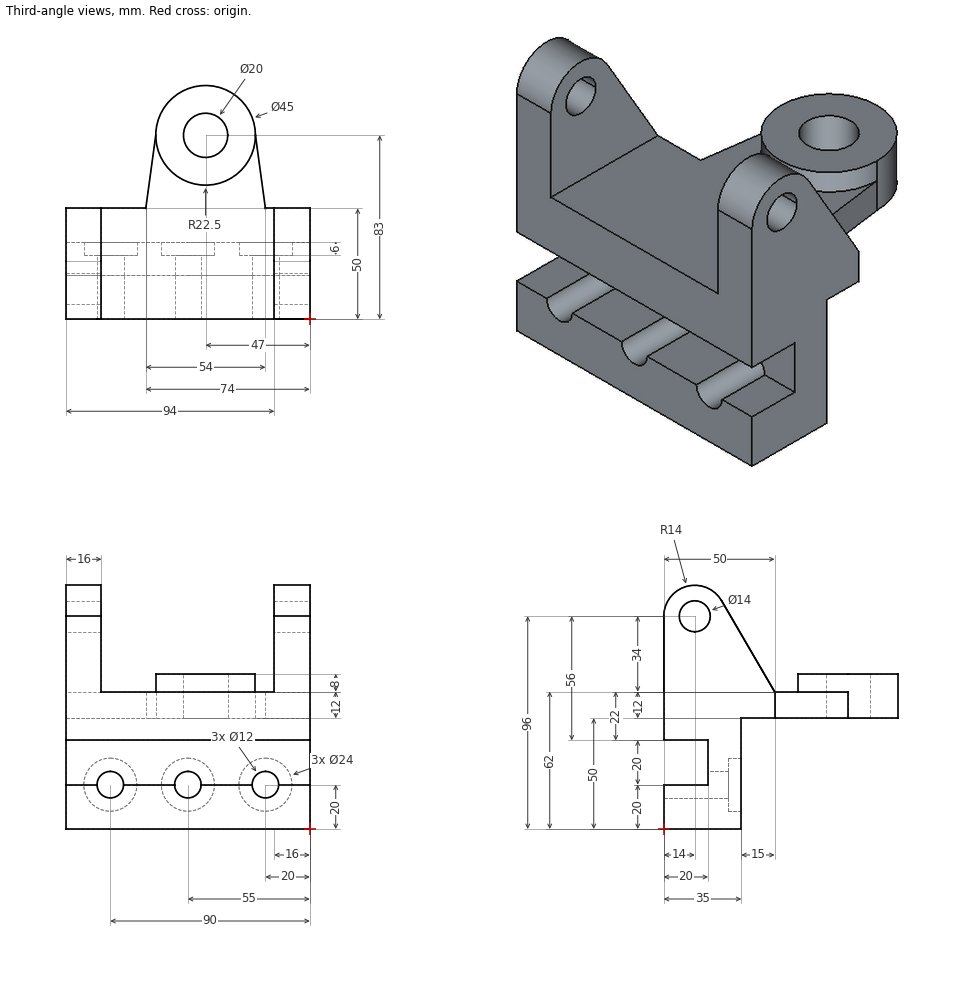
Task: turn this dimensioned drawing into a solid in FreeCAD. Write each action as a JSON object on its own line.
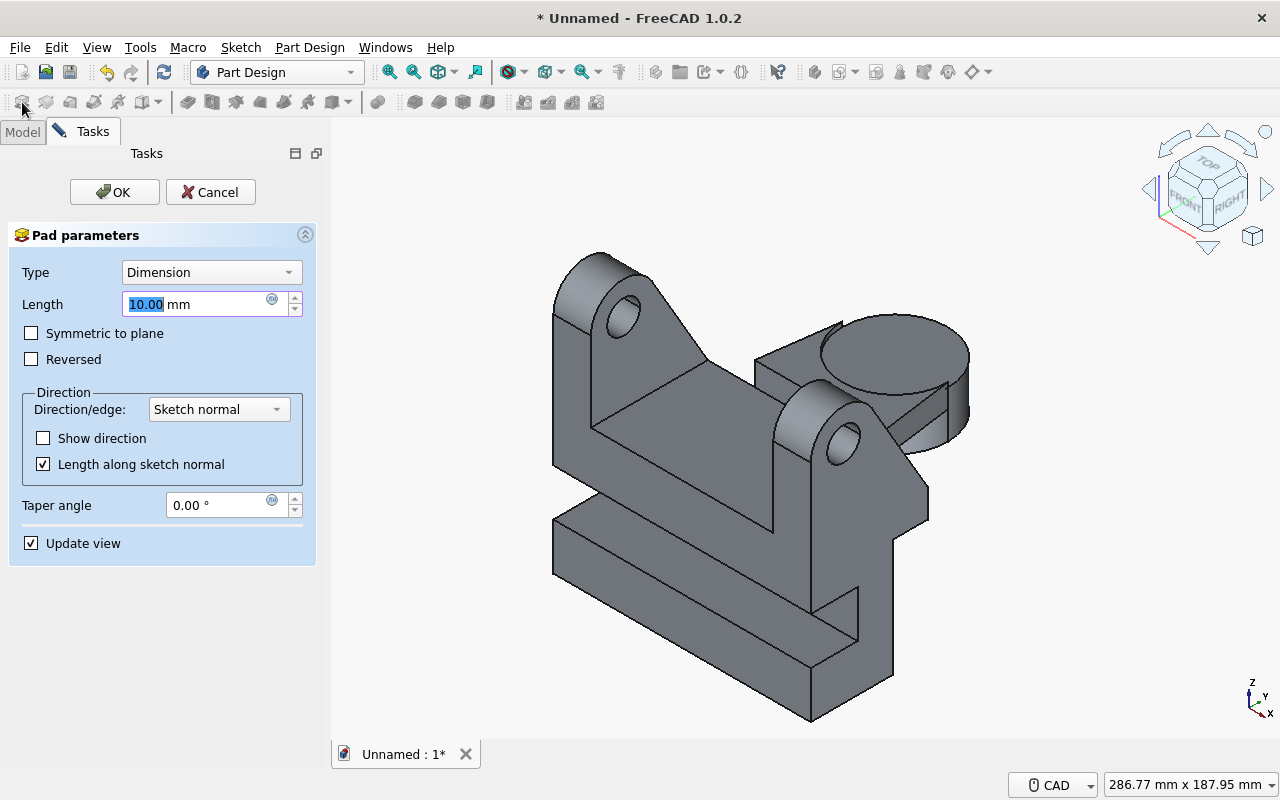
{"action": "type", "text": "12"}
{"action": "key", "text": "Tab"}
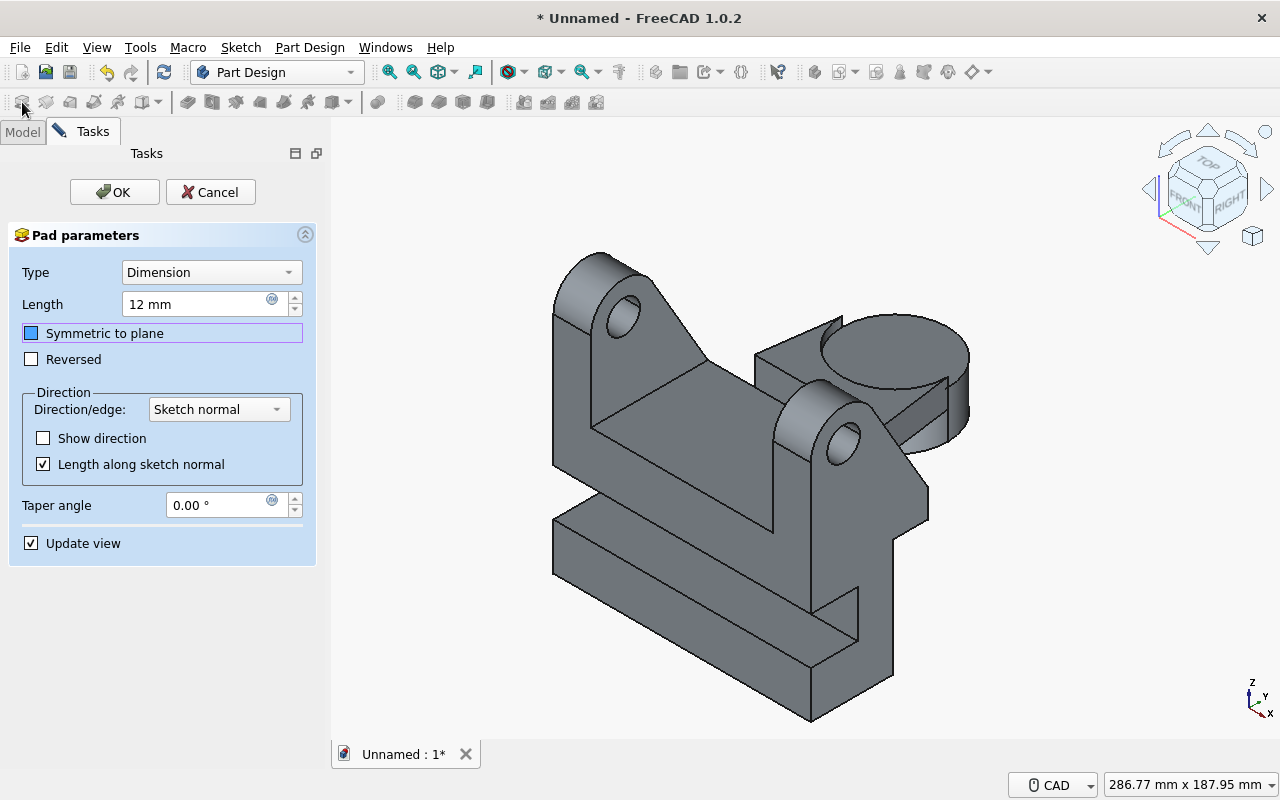
{"action": "left_click", "coordinate": [30, 359]}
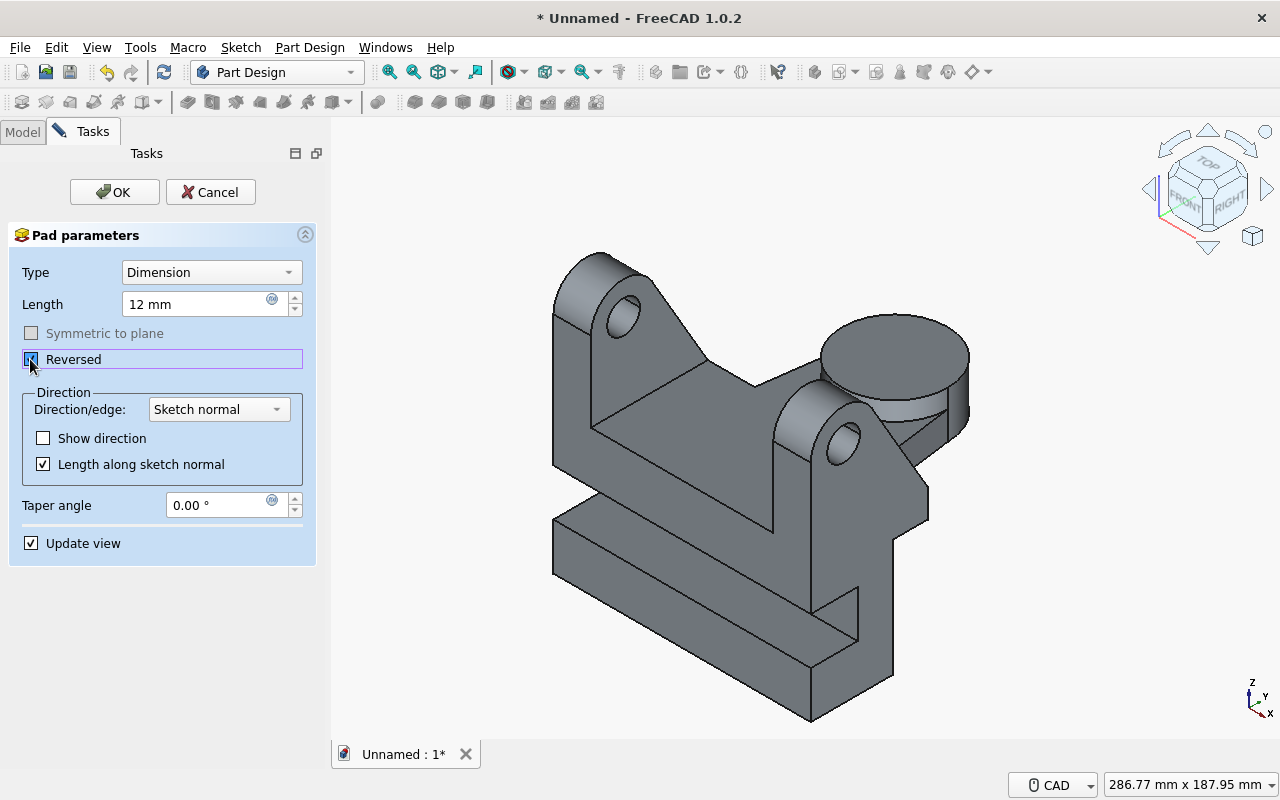
{"action": "left_click", "coordinate": [115, 192]}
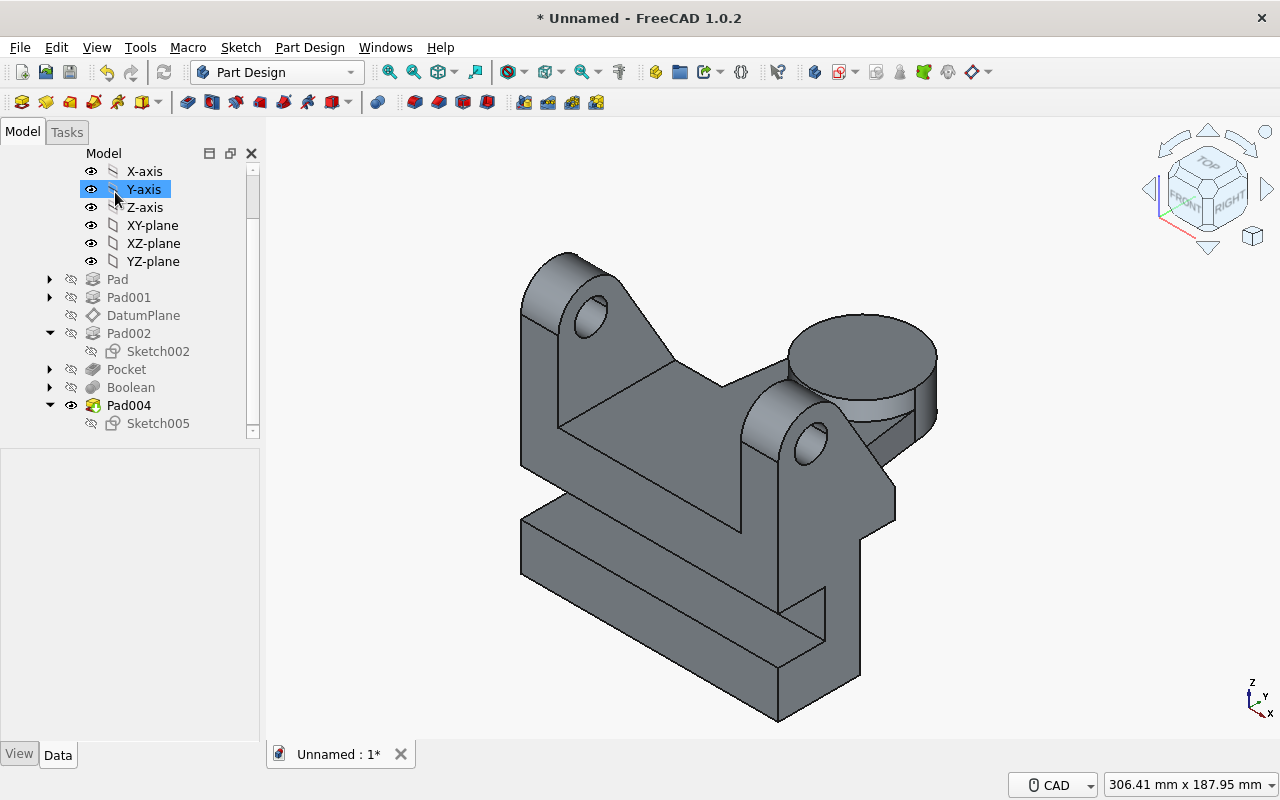
{"action": "left_click", "coordinate": [863, 356]}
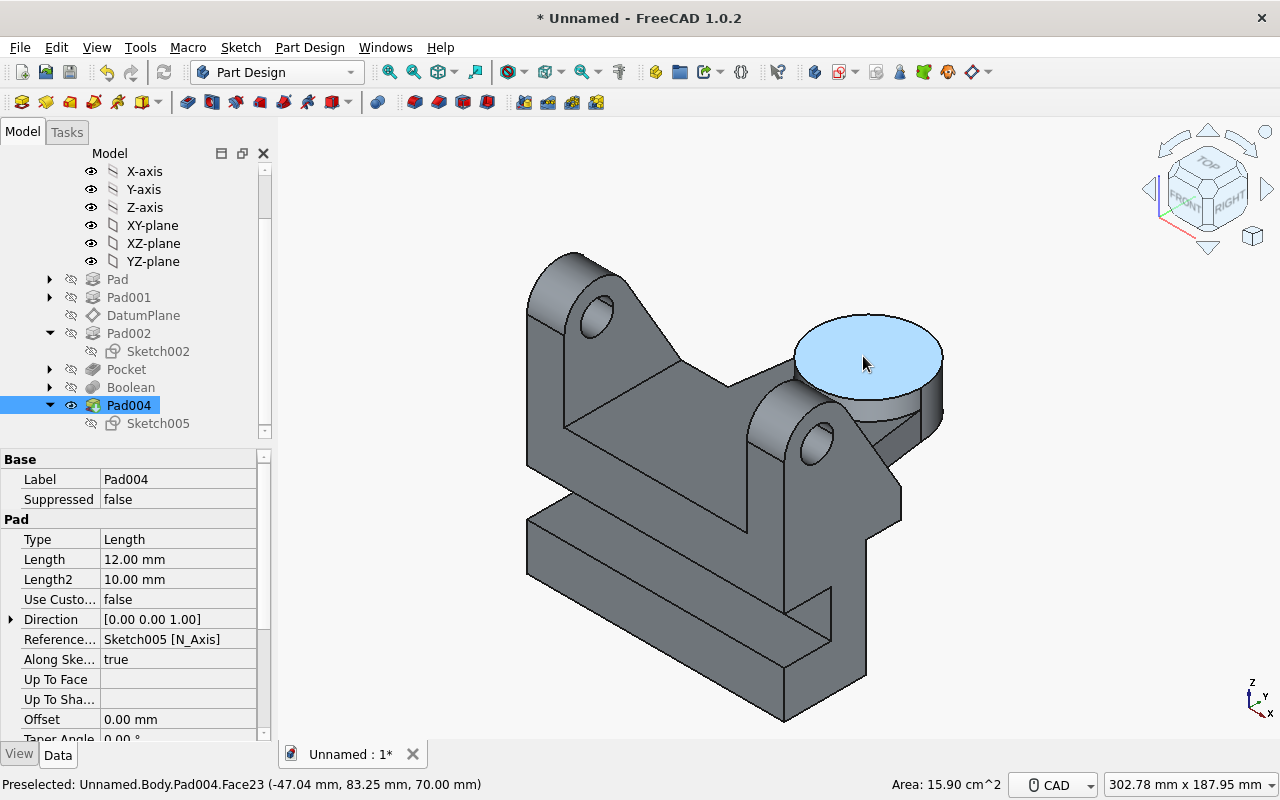
{"action": "left_click", "coordinate": [840, 72]}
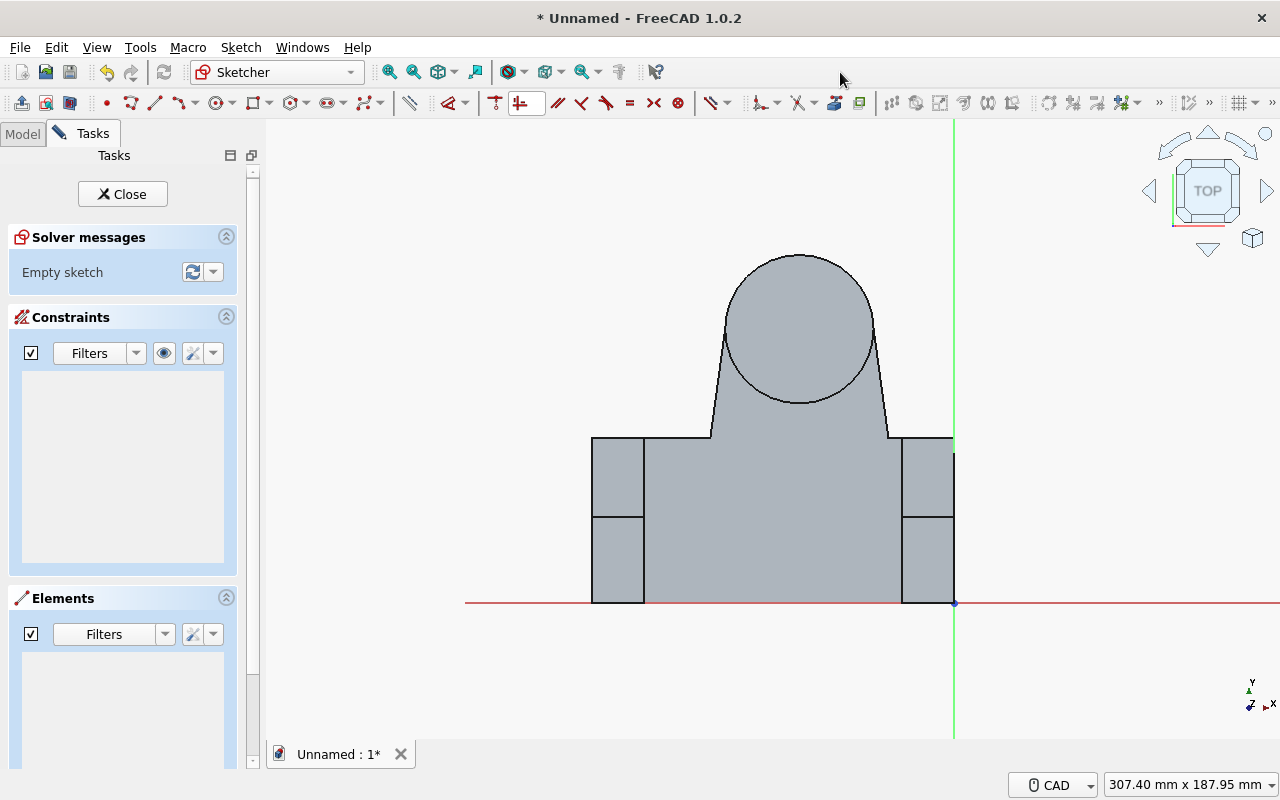
{"action": "left_click", "coordinate": [70, 104]}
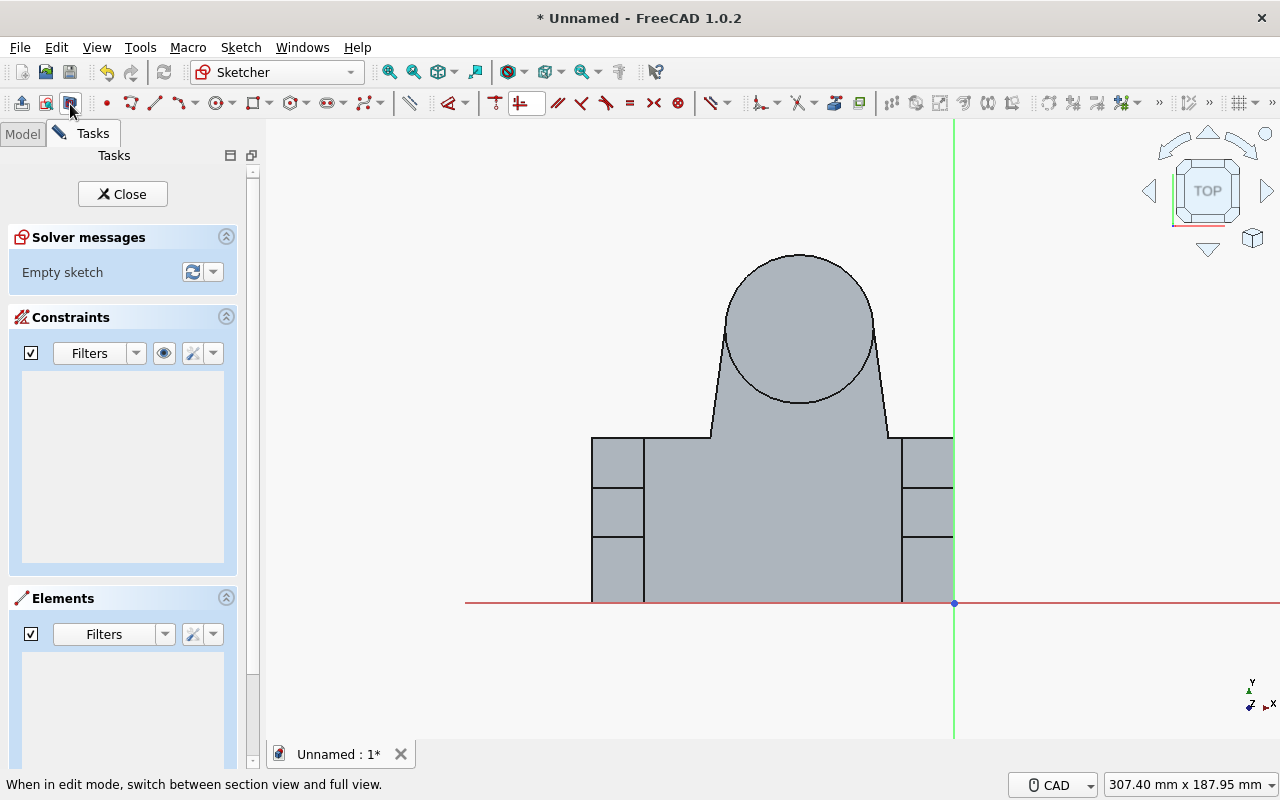
{"action": "scroll", "coordinate": [818, 309], "scroll_direction": "up", "scroll_amount": 9}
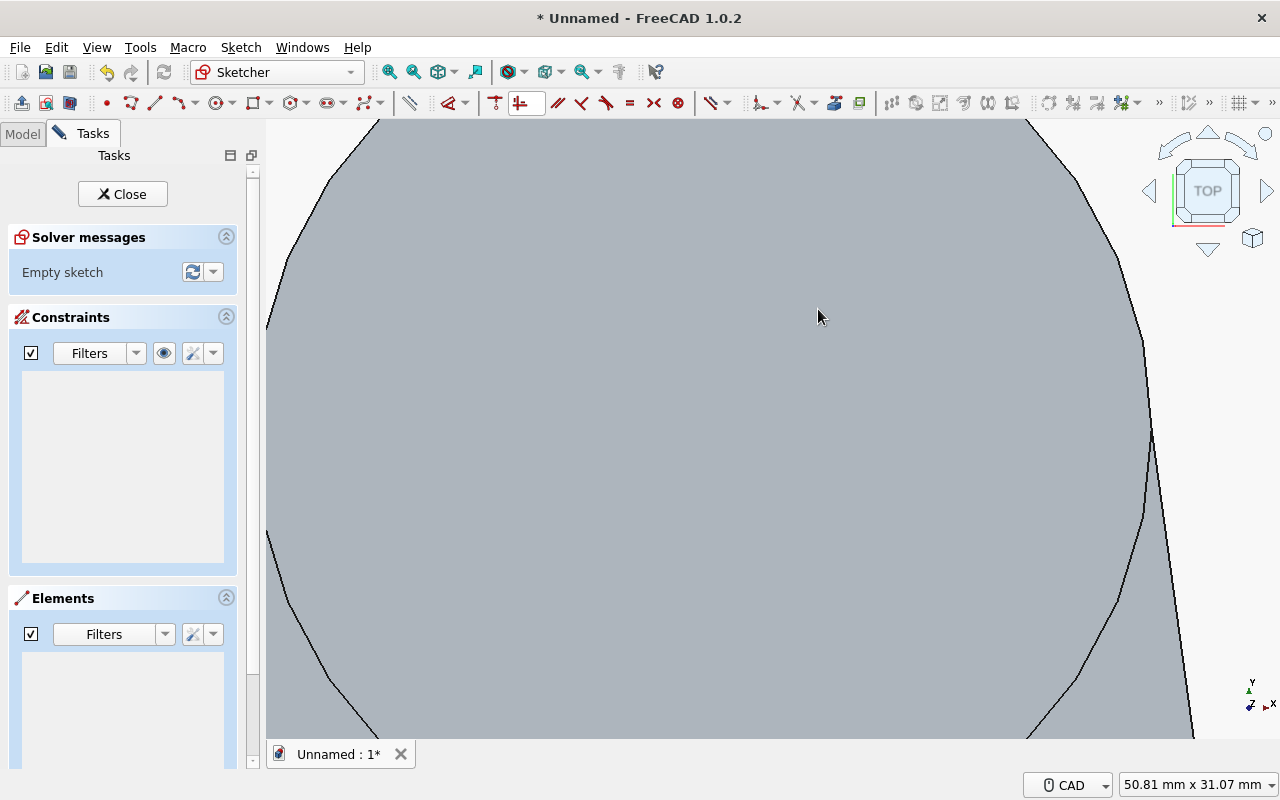
{"action": "left_click", "coordinate": [216, 104]}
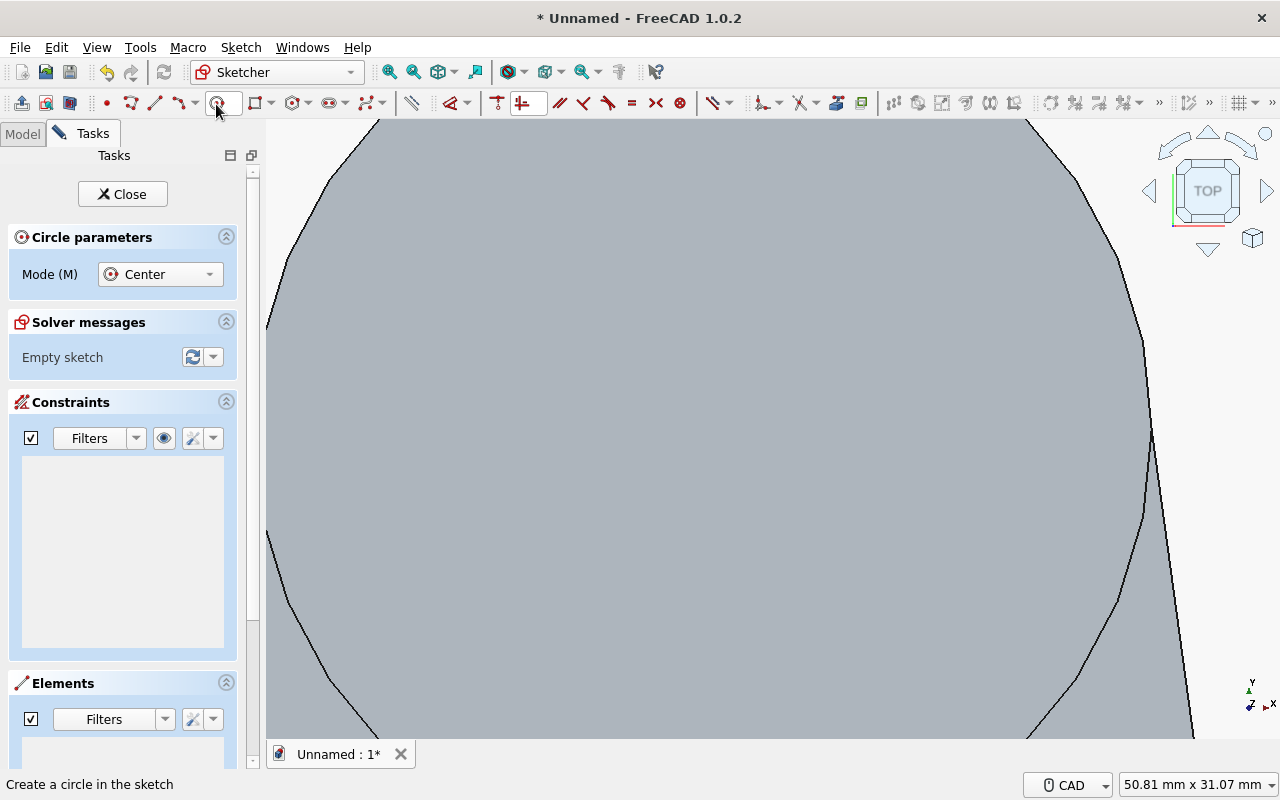
{"action": "left_click", "coordinate": [703, 430]}
{"action": "mouse_move", "coordinate": [844, 289]}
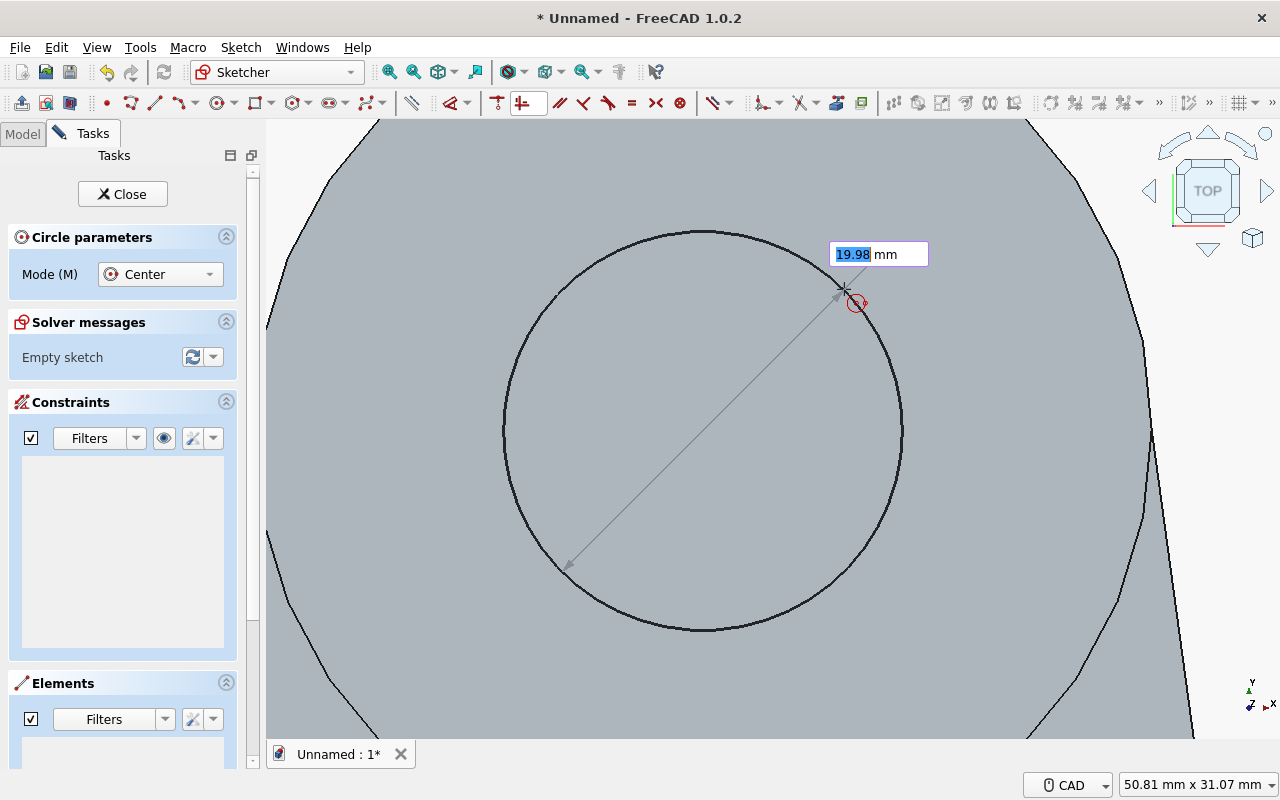
{"action": "type", "text": "20"}
{"action": "key", "text": "Return"}
{"action": "key", "text": "Escape"}